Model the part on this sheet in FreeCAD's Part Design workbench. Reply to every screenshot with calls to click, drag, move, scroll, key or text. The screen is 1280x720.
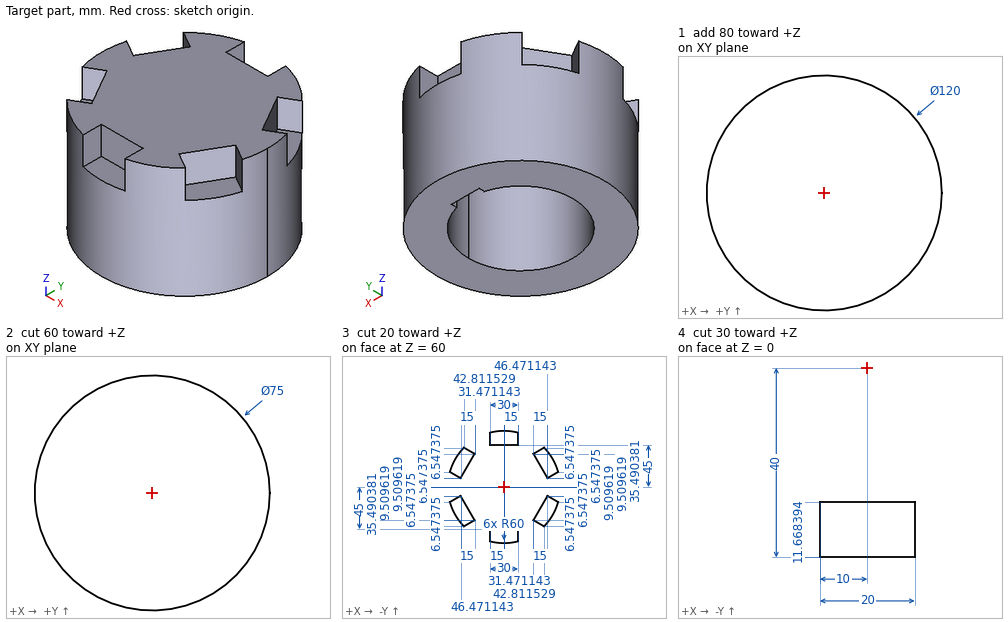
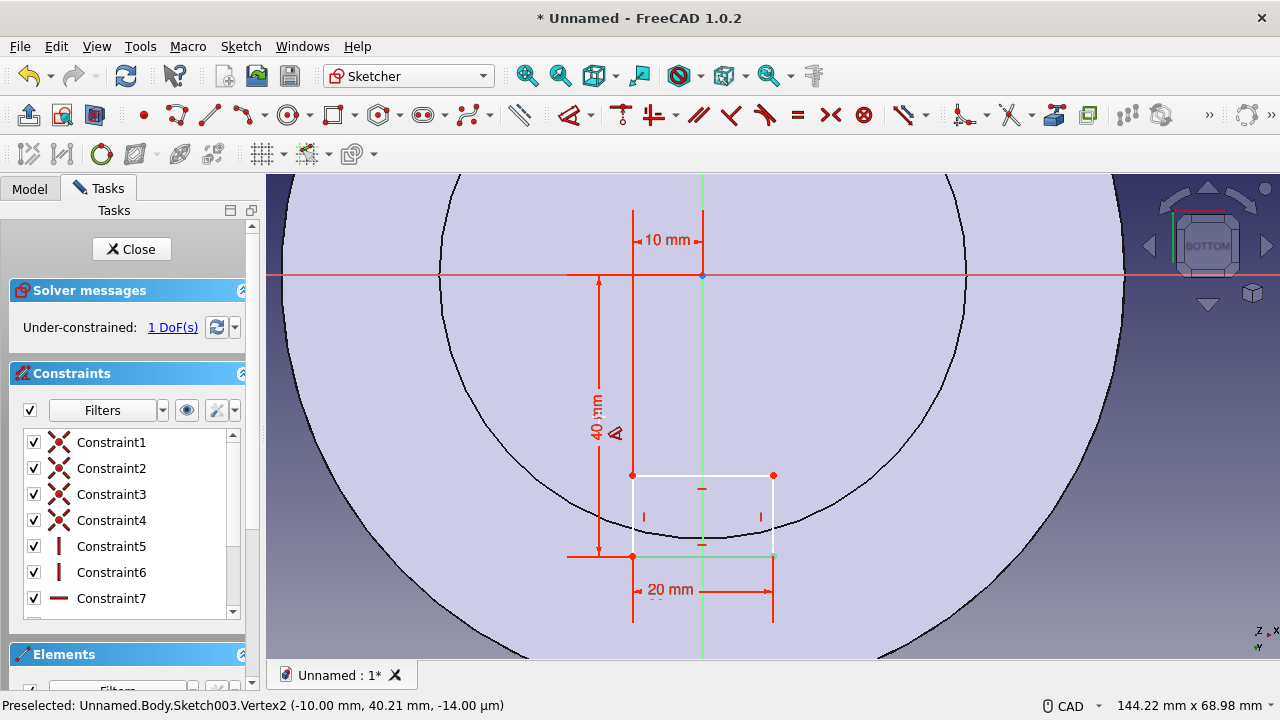
click(633, 500)
click(599, 516)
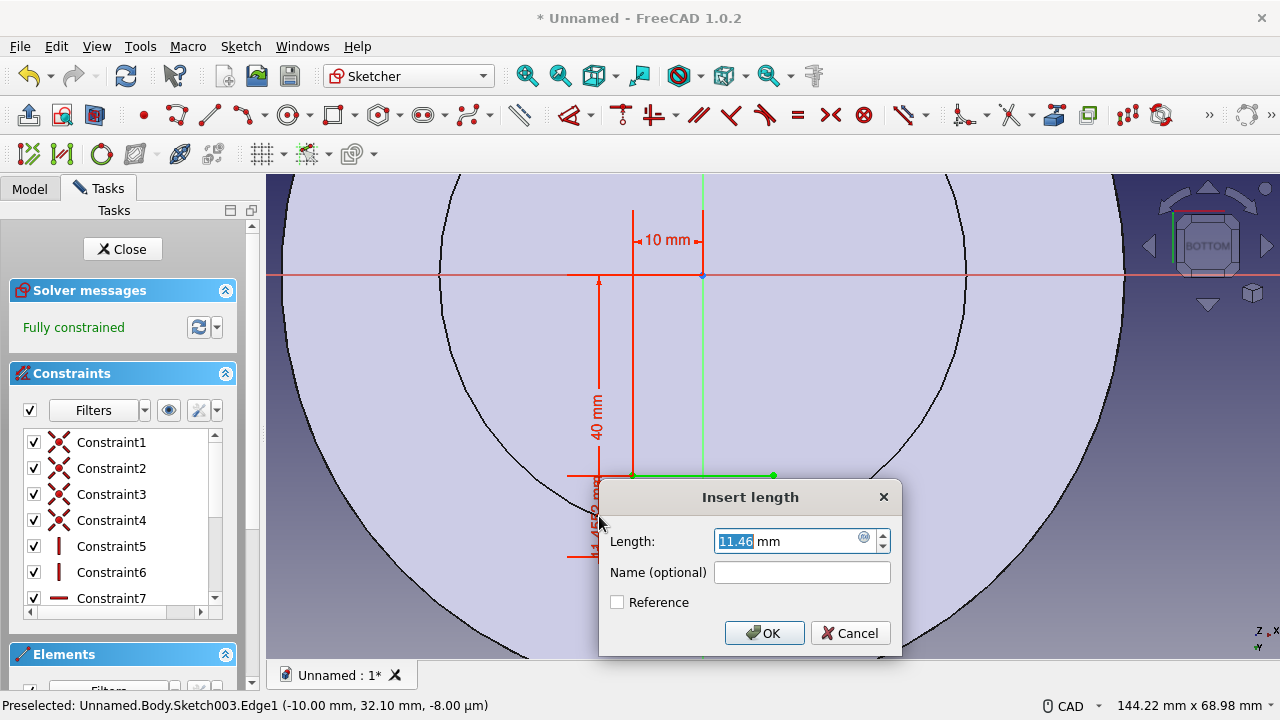
text(11.668394)
key(Return)
key(Escape)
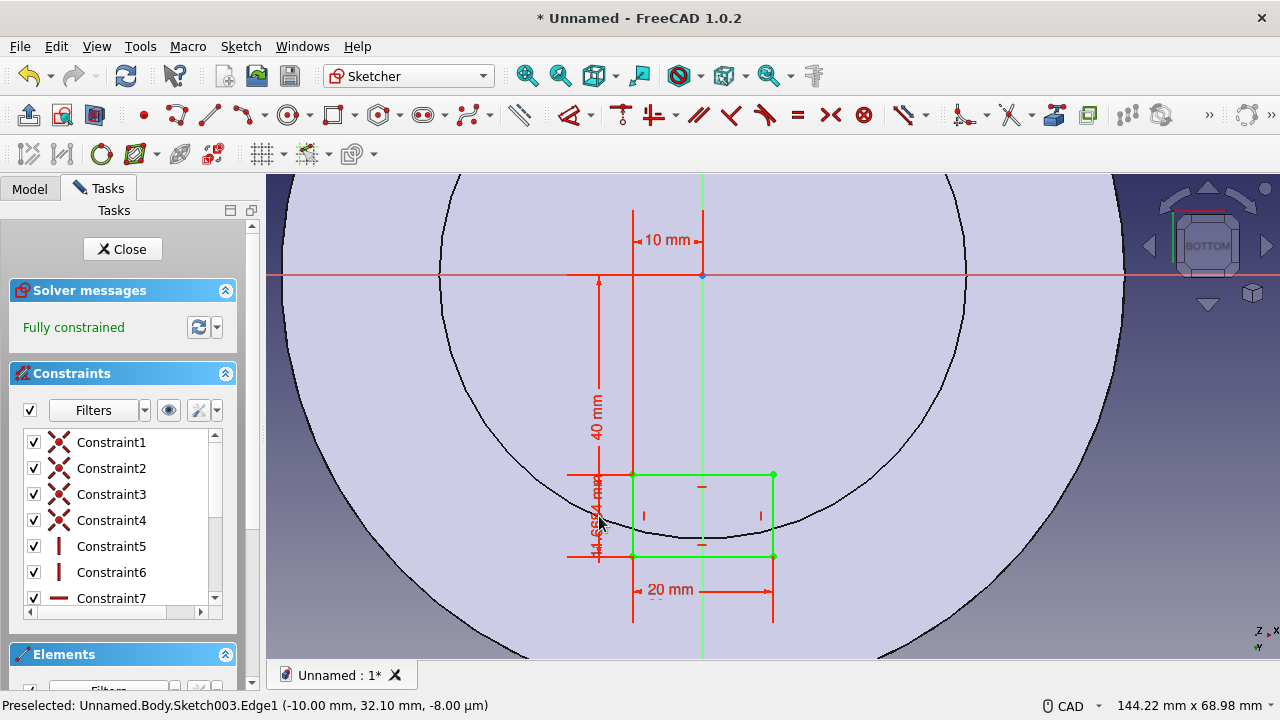
click(123, 249)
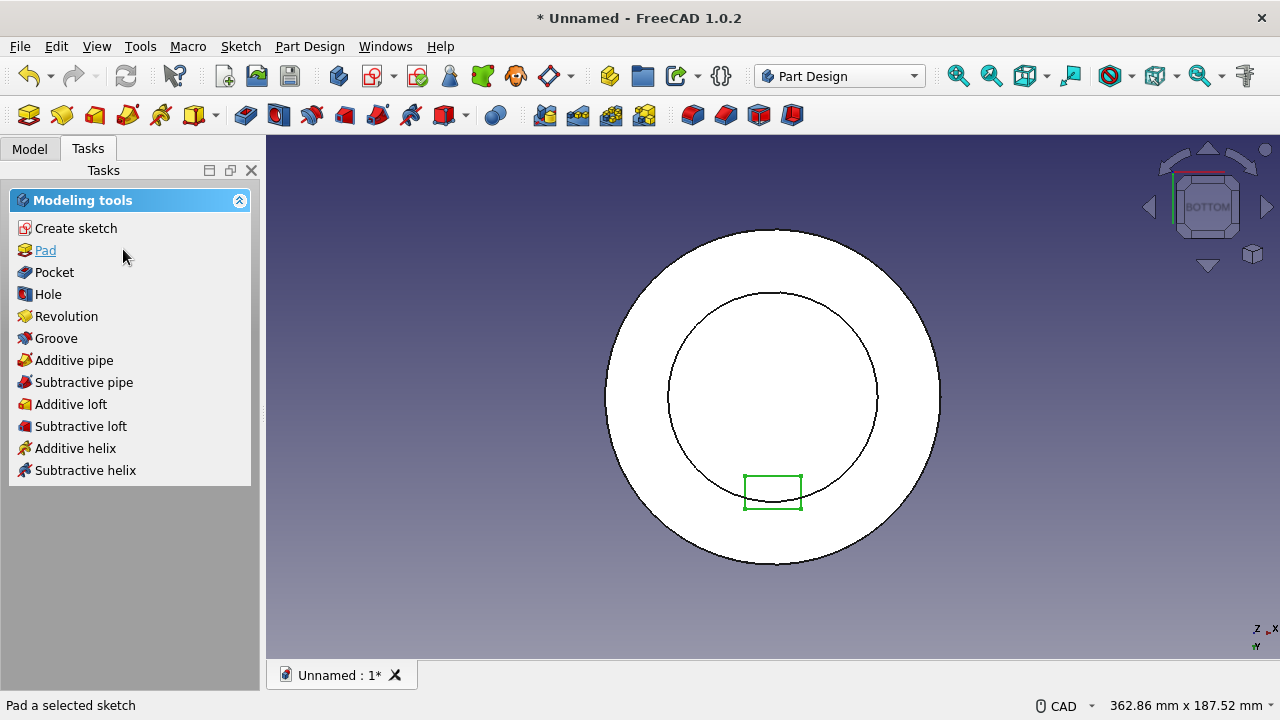
click(246, 116)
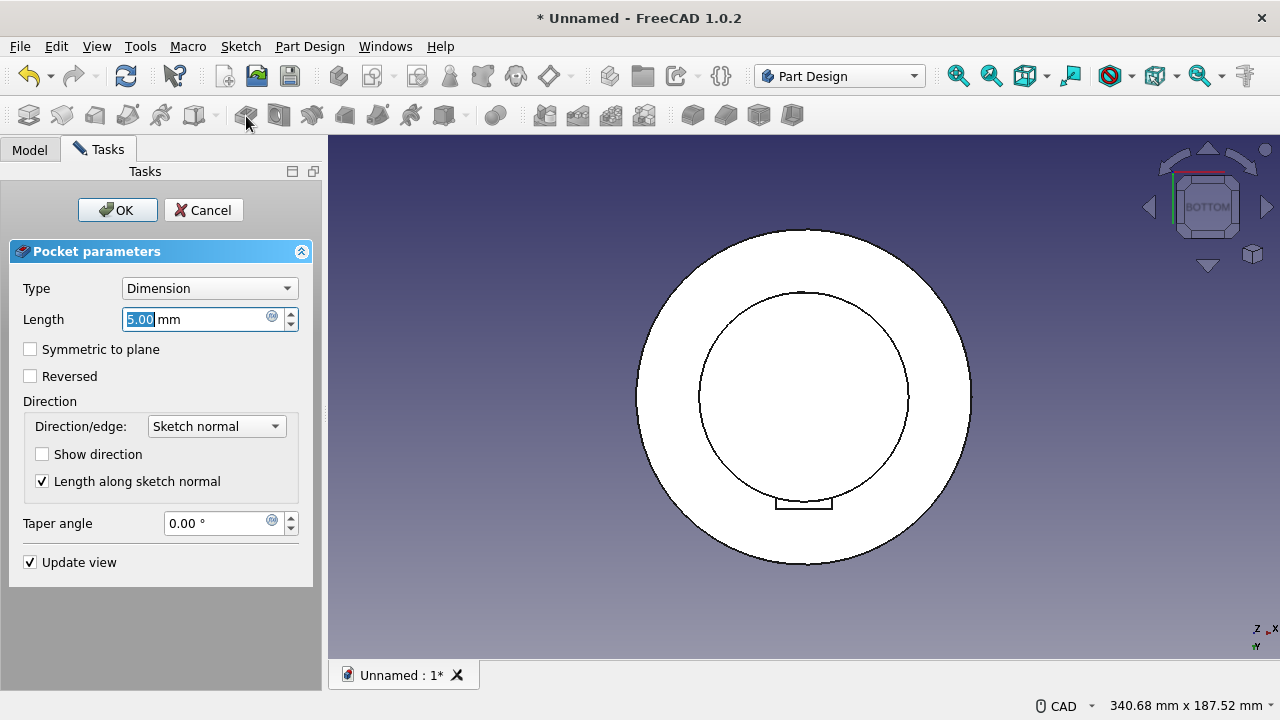
text(30)
key(Tab)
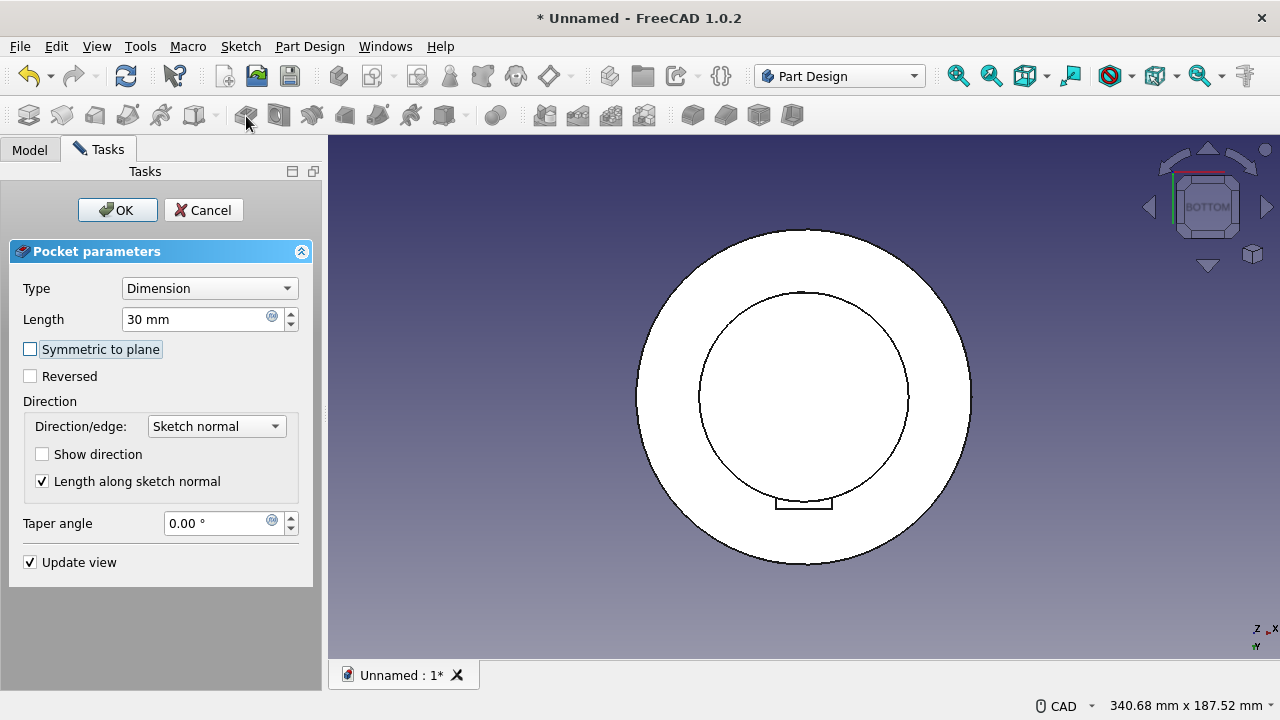
click(118, 210)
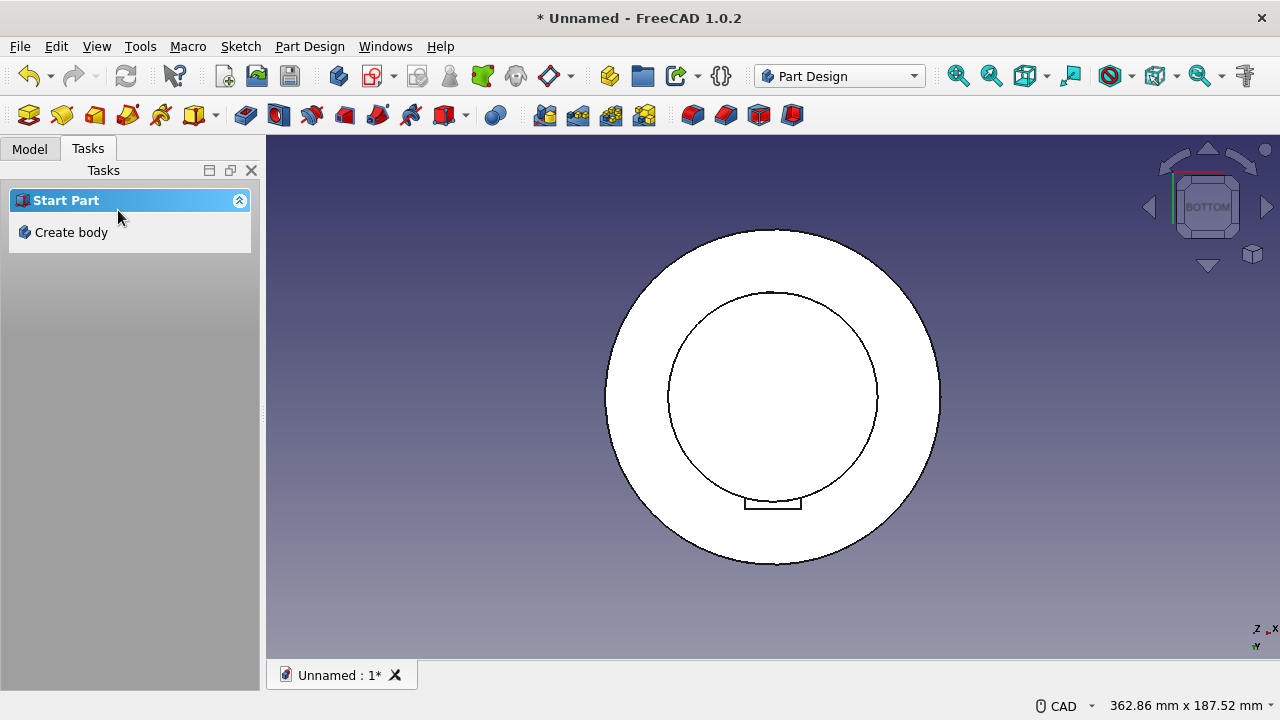
key(0)